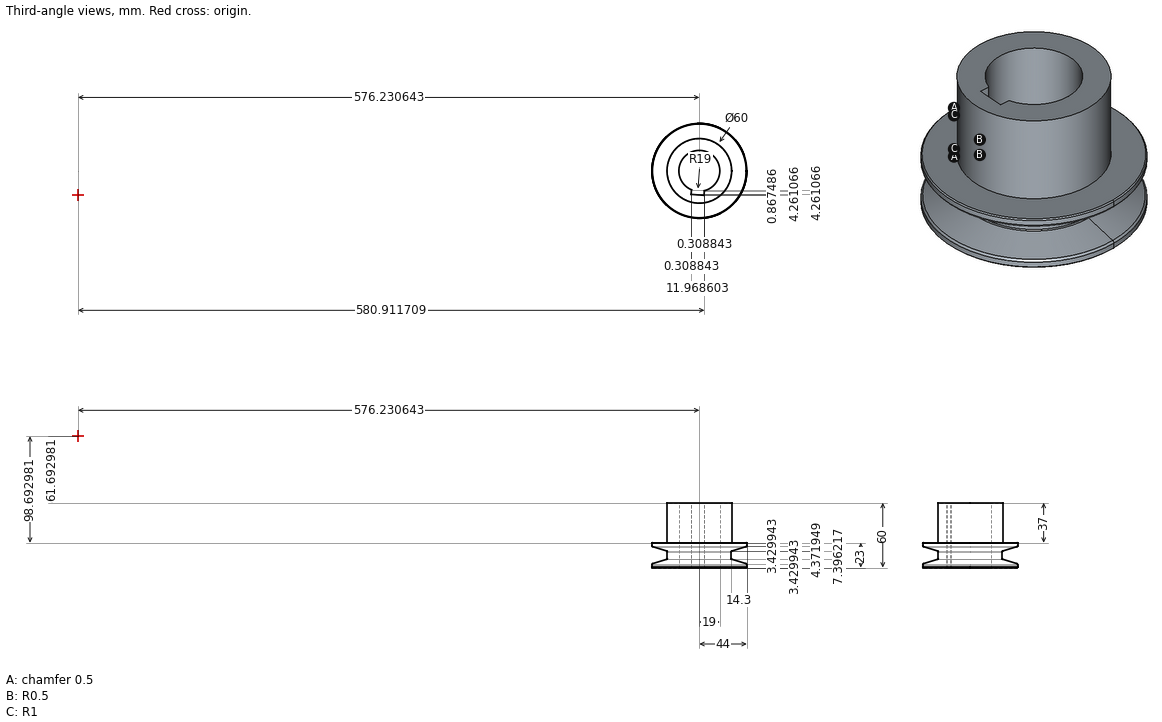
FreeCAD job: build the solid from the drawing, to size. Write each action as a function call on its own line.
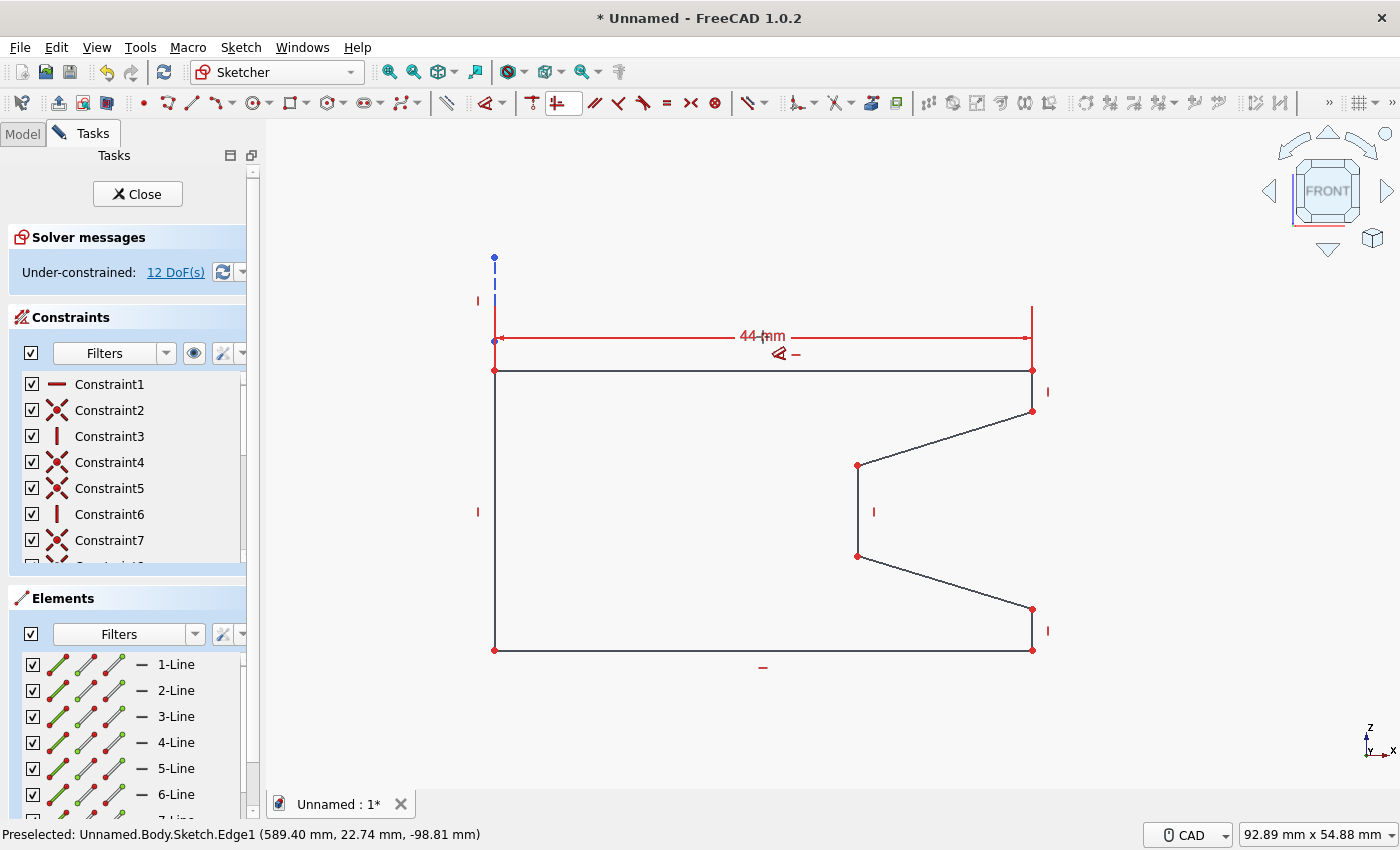
click(871, 651)
click(763, 685)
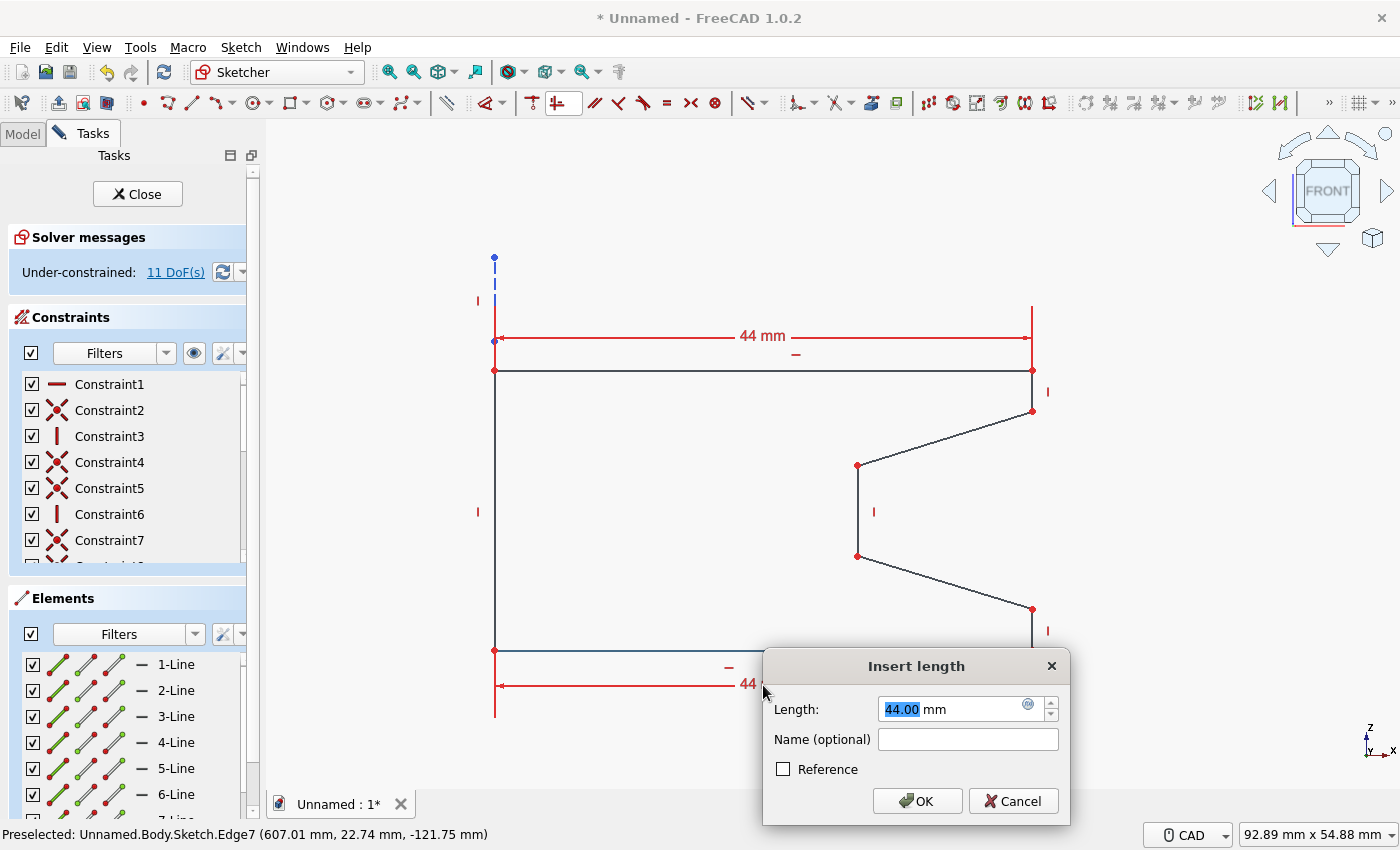
text(44)
key(Return)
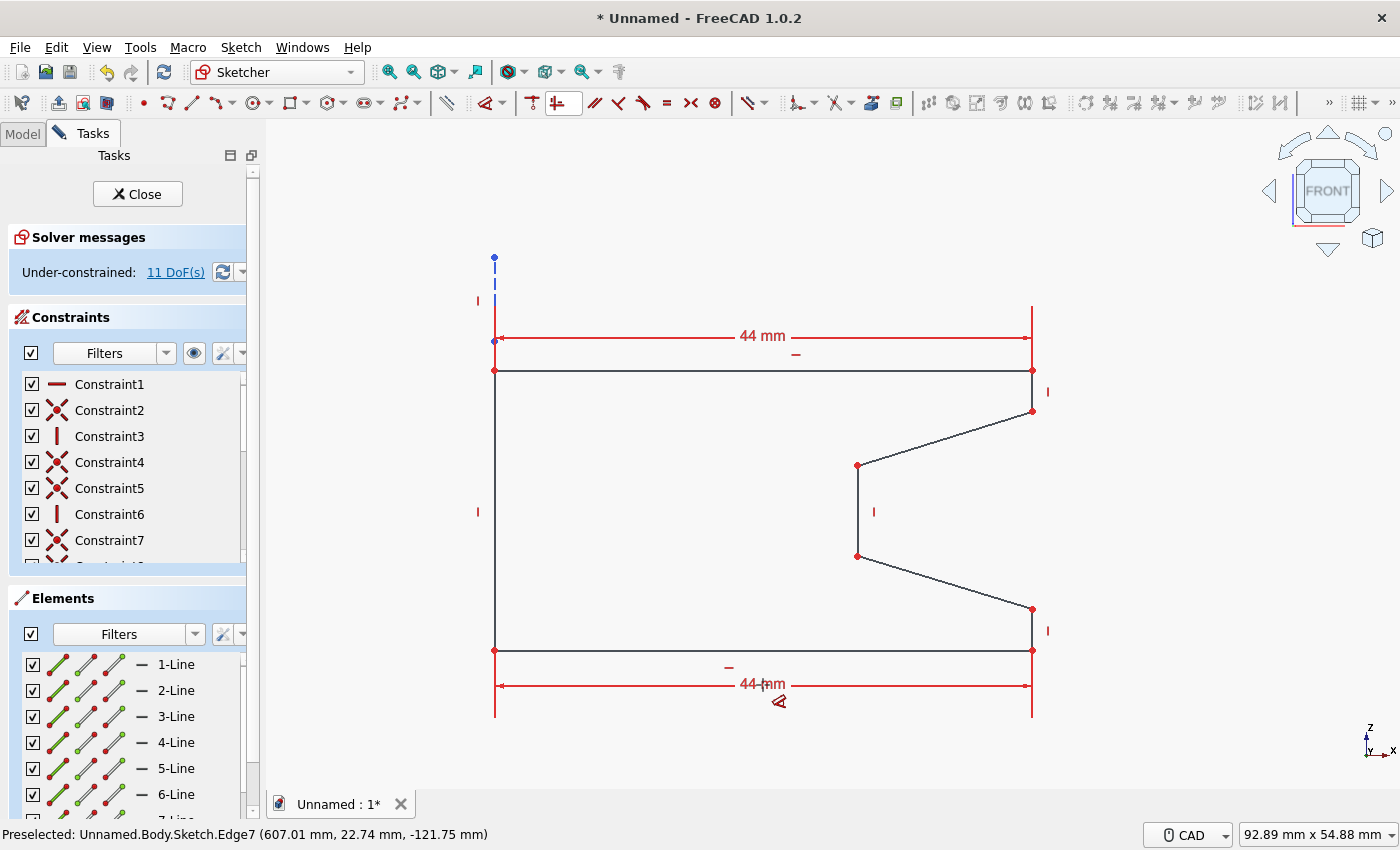
click(495, 567)
click(461, 511)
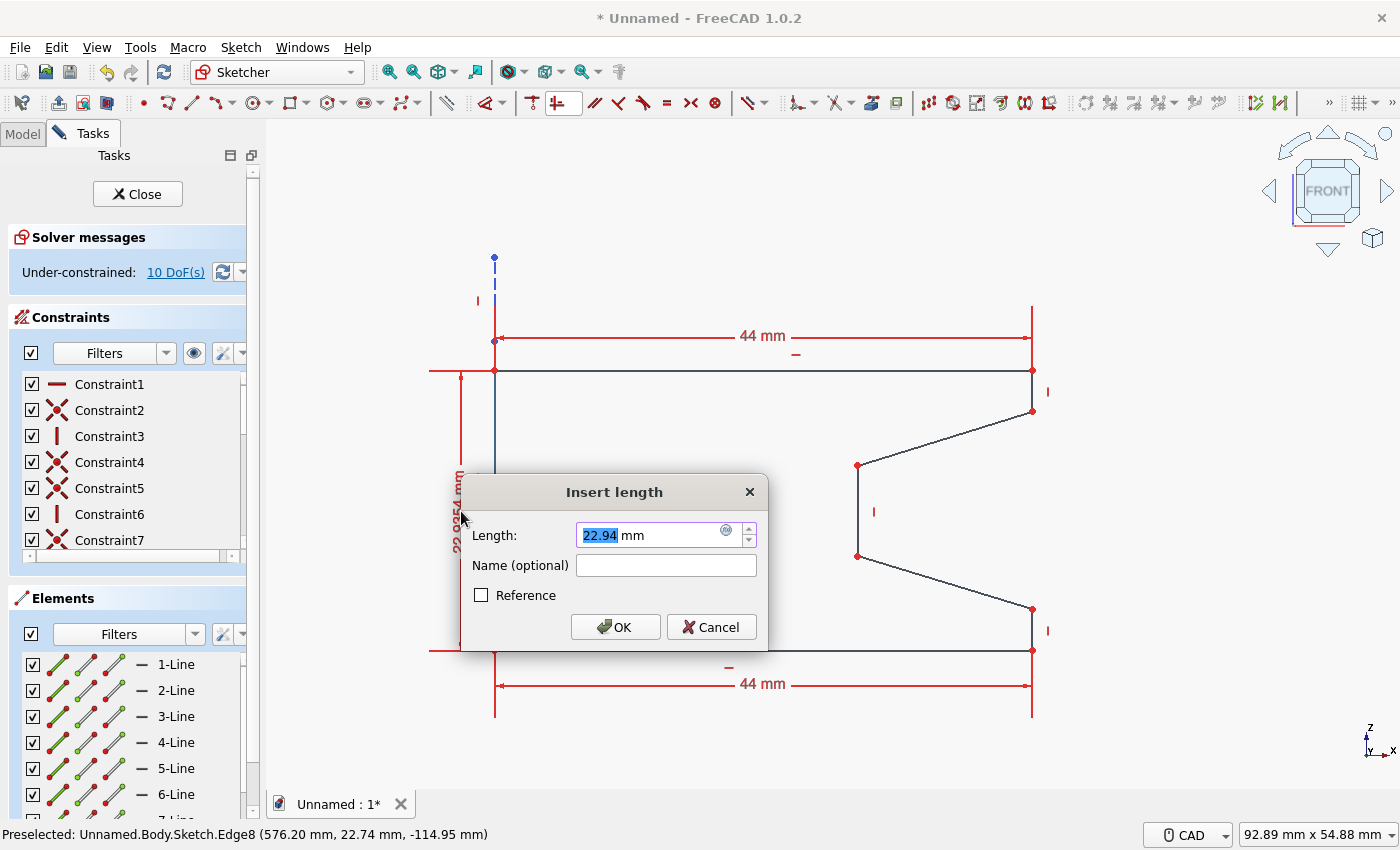
text(23)
key(Return)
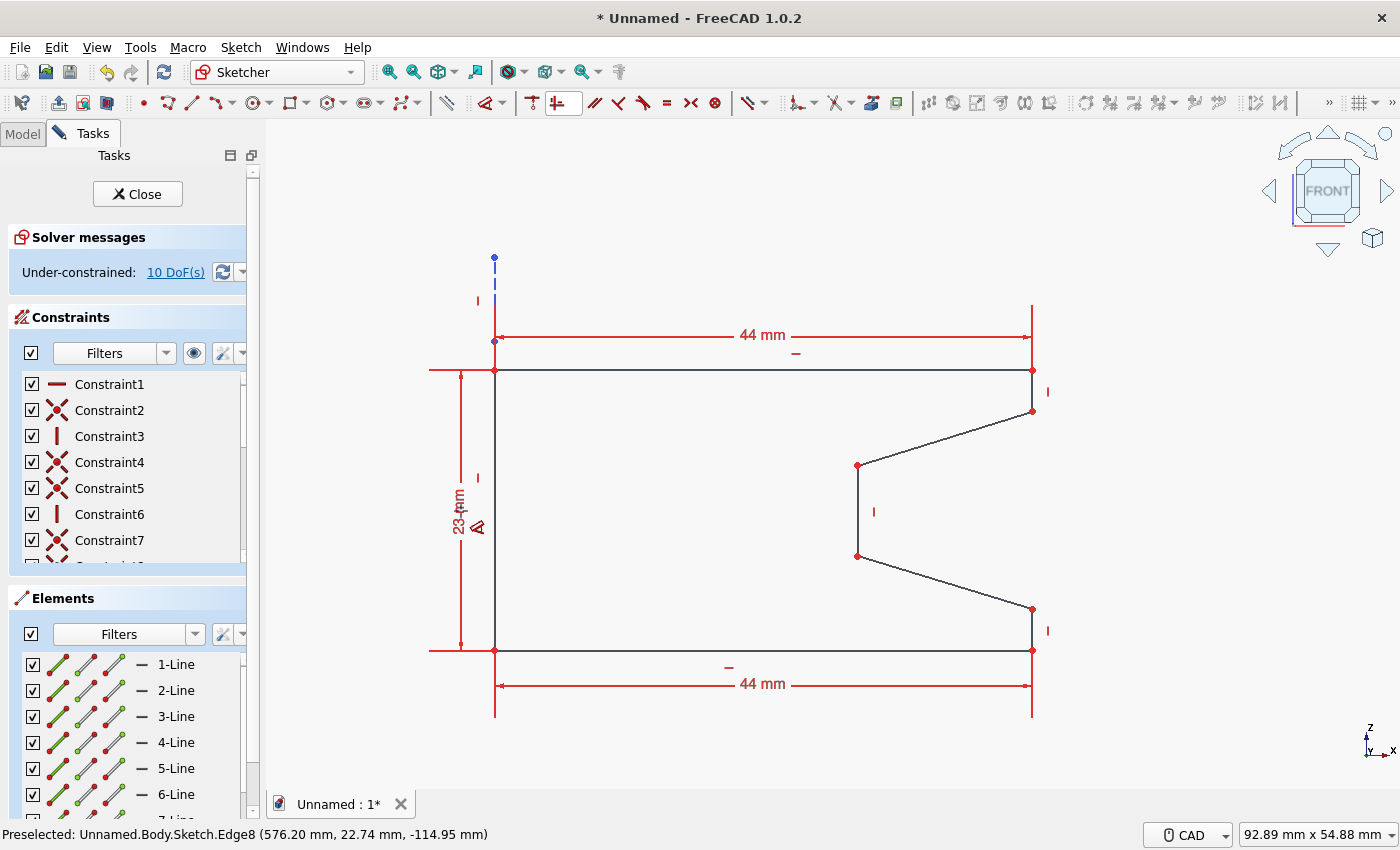
click(980, 428)
click(945, 500)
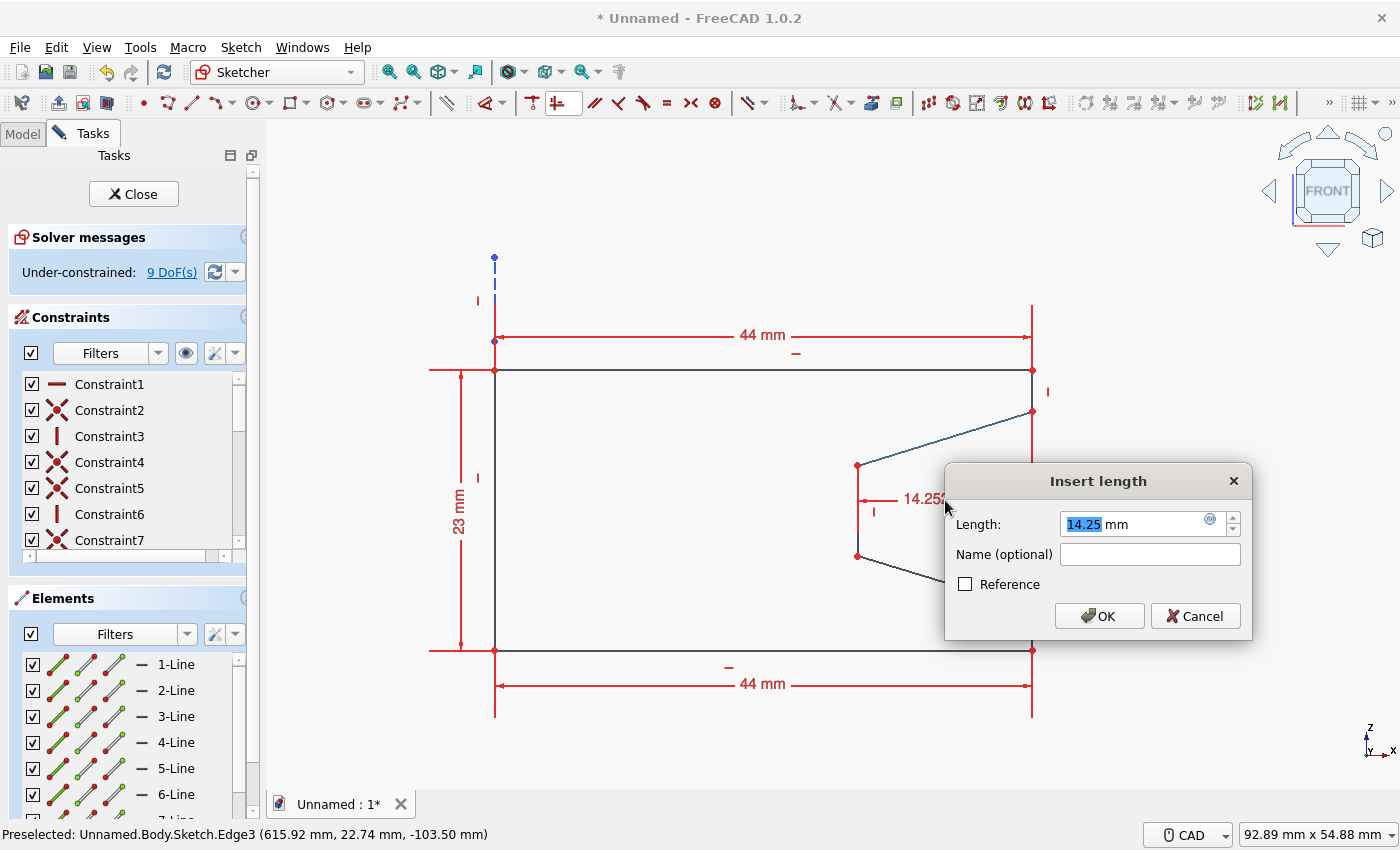
text(14.3)
key(Return)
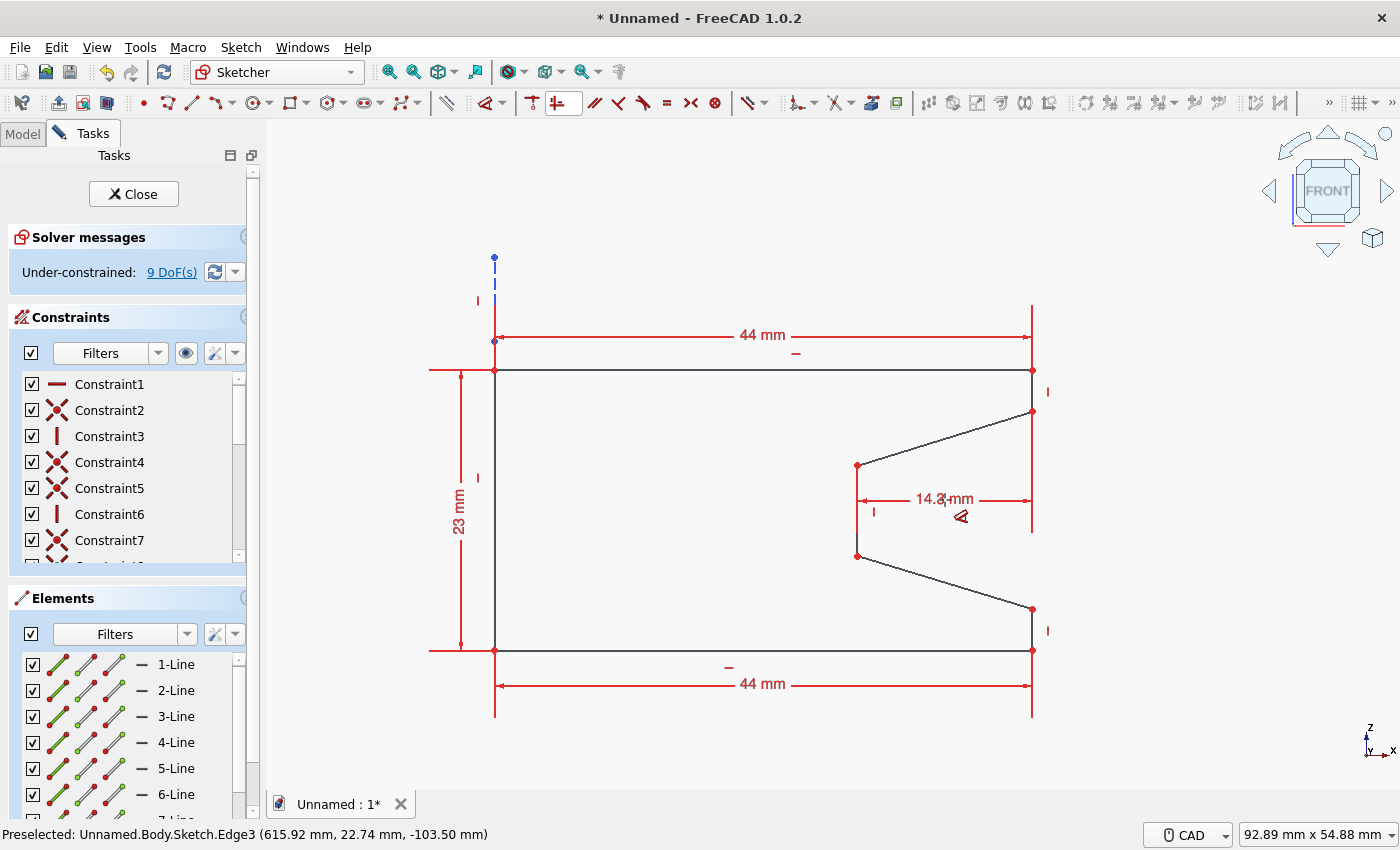
click(1032, 383)
click(1066, 391)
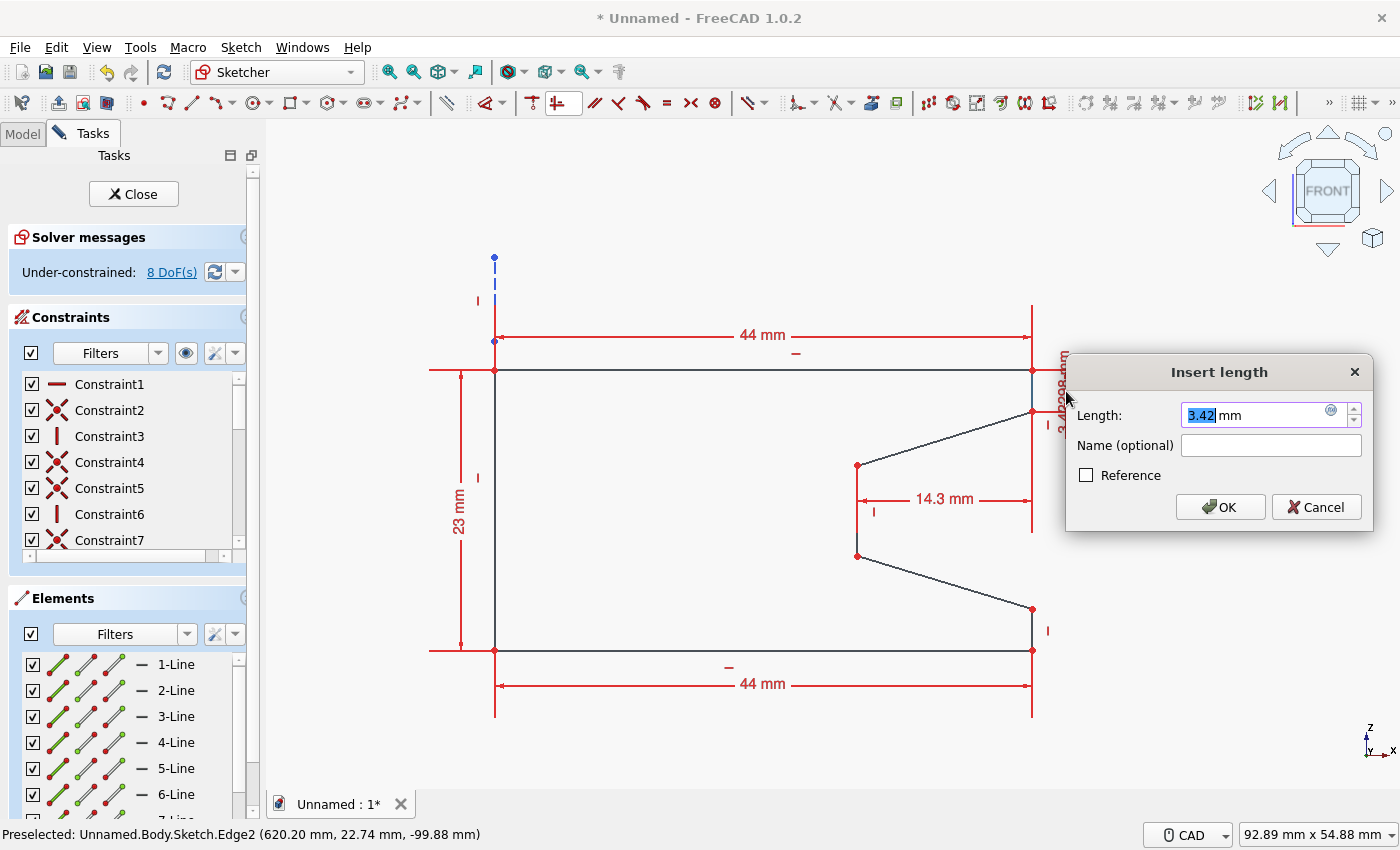
text(3.429943)
key(Return)